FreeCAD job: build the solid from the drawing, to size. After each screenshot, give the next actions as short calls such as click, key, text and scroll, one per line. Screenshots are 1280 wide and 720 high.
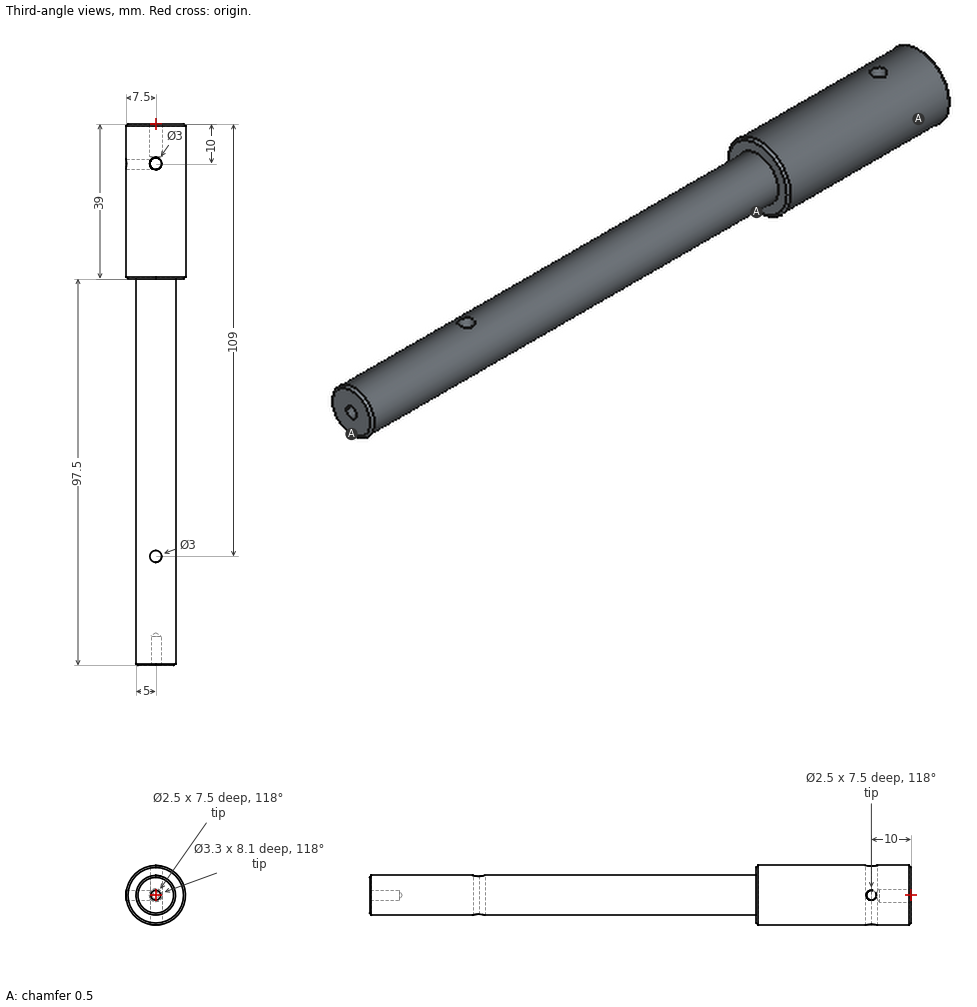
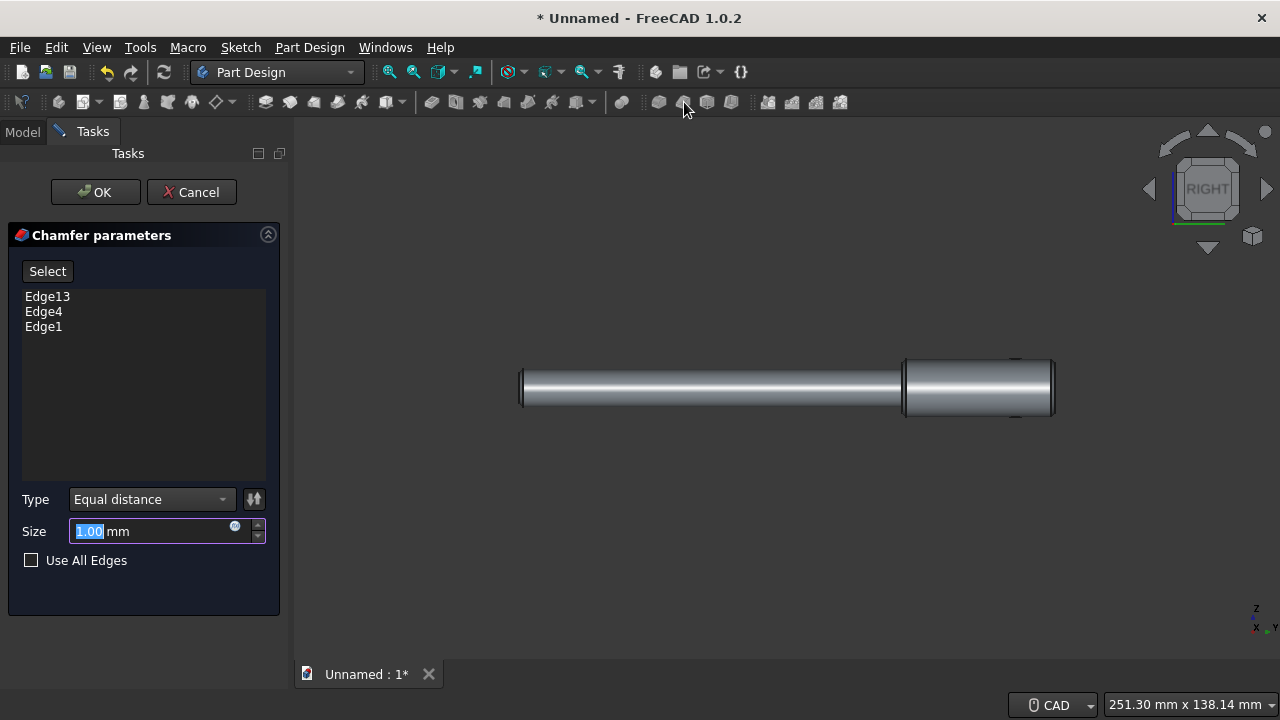
text(0.5)
key(Tab)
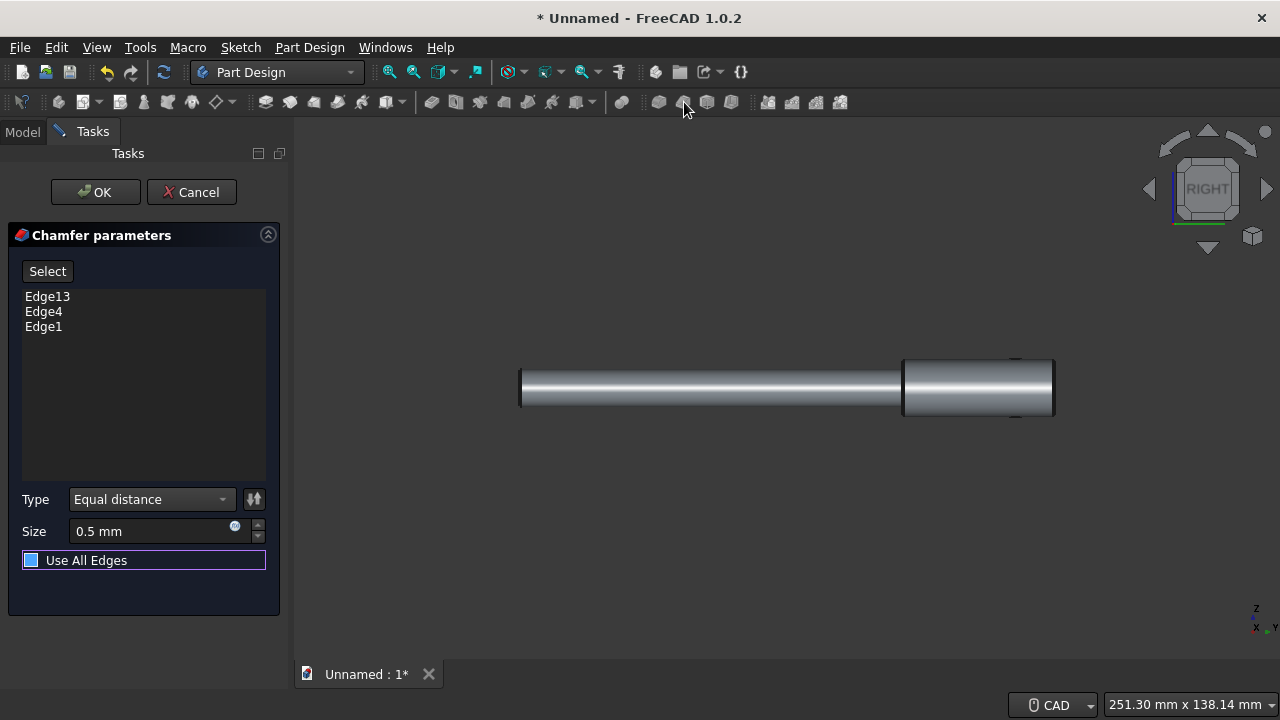
click(96, 192)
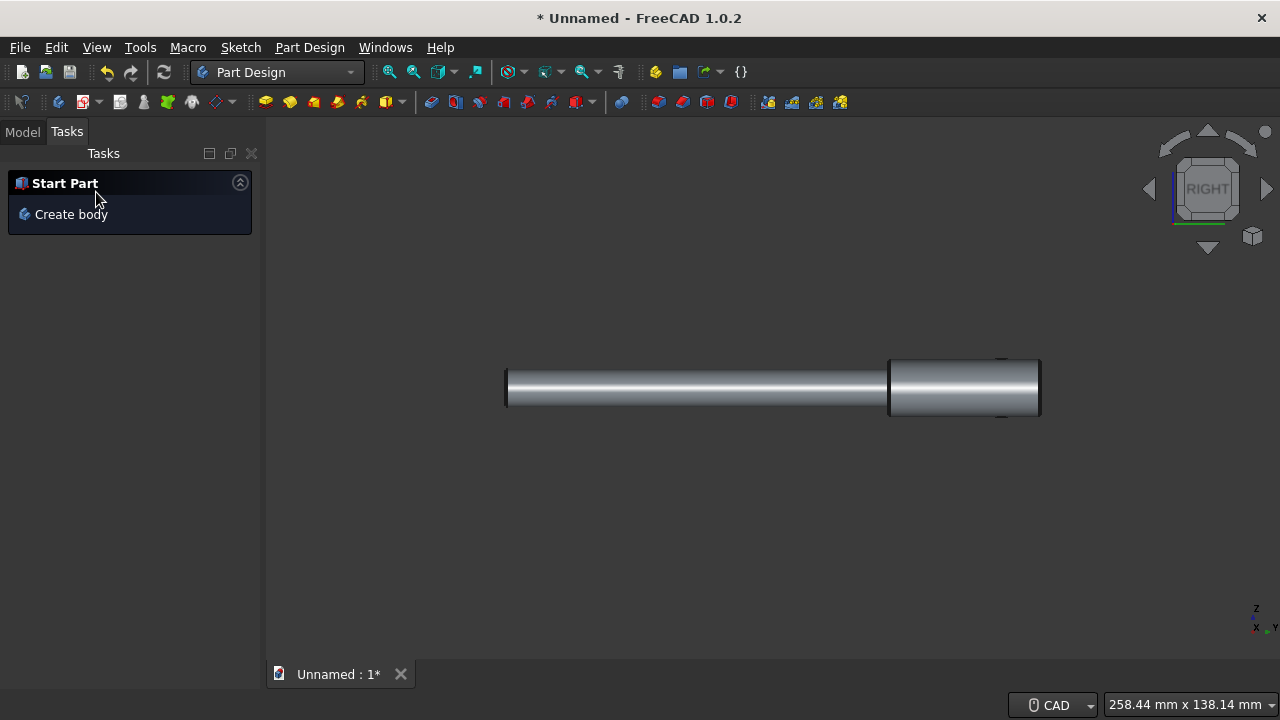
click(23, 131)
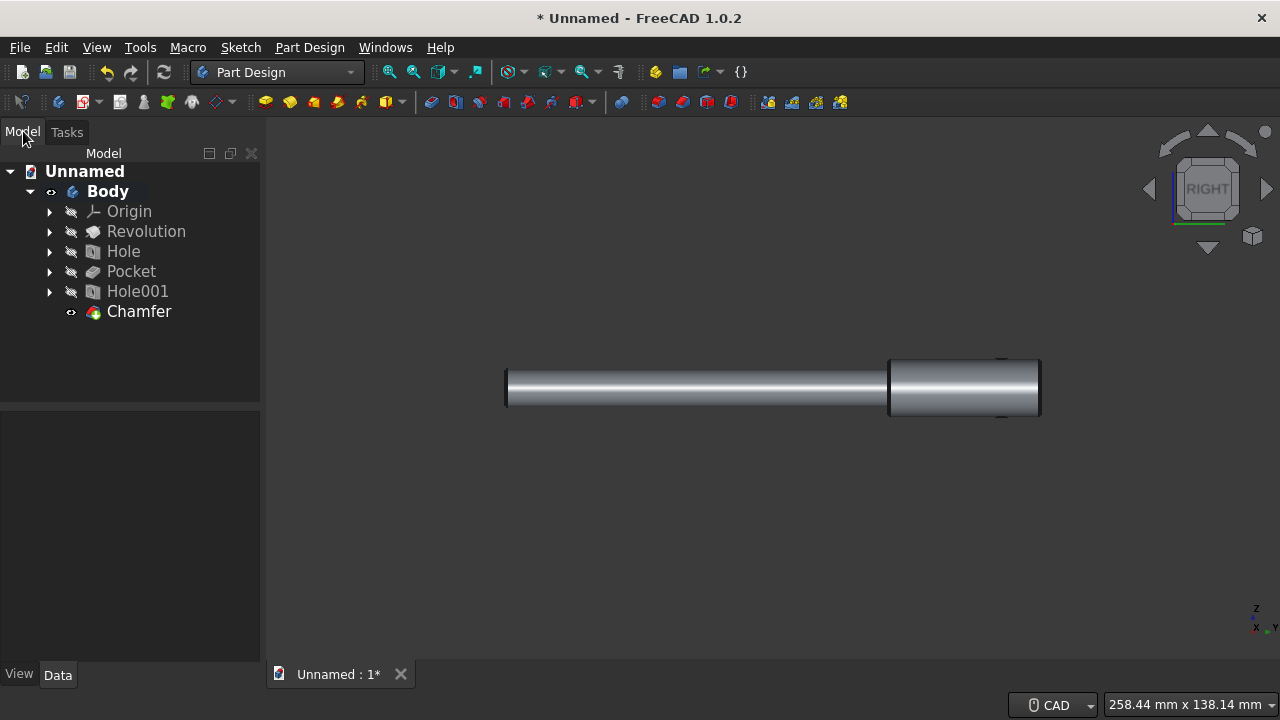
click(50, 212)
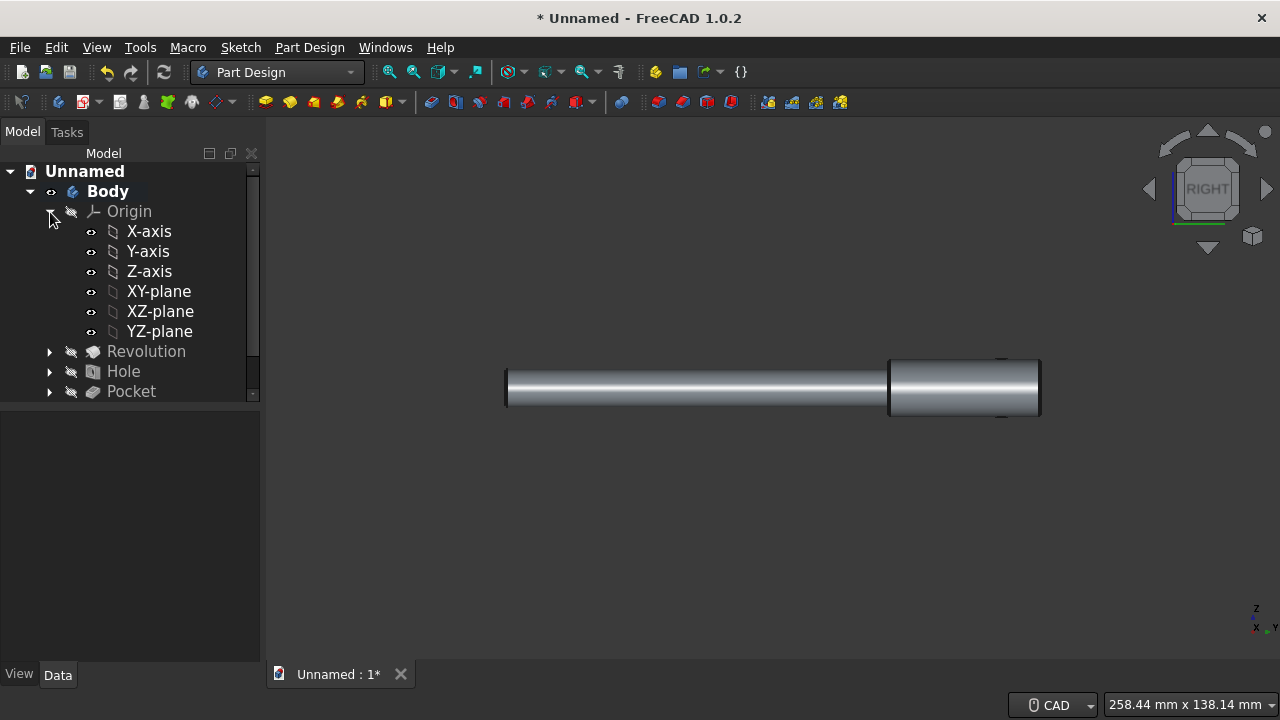
click(136, 332)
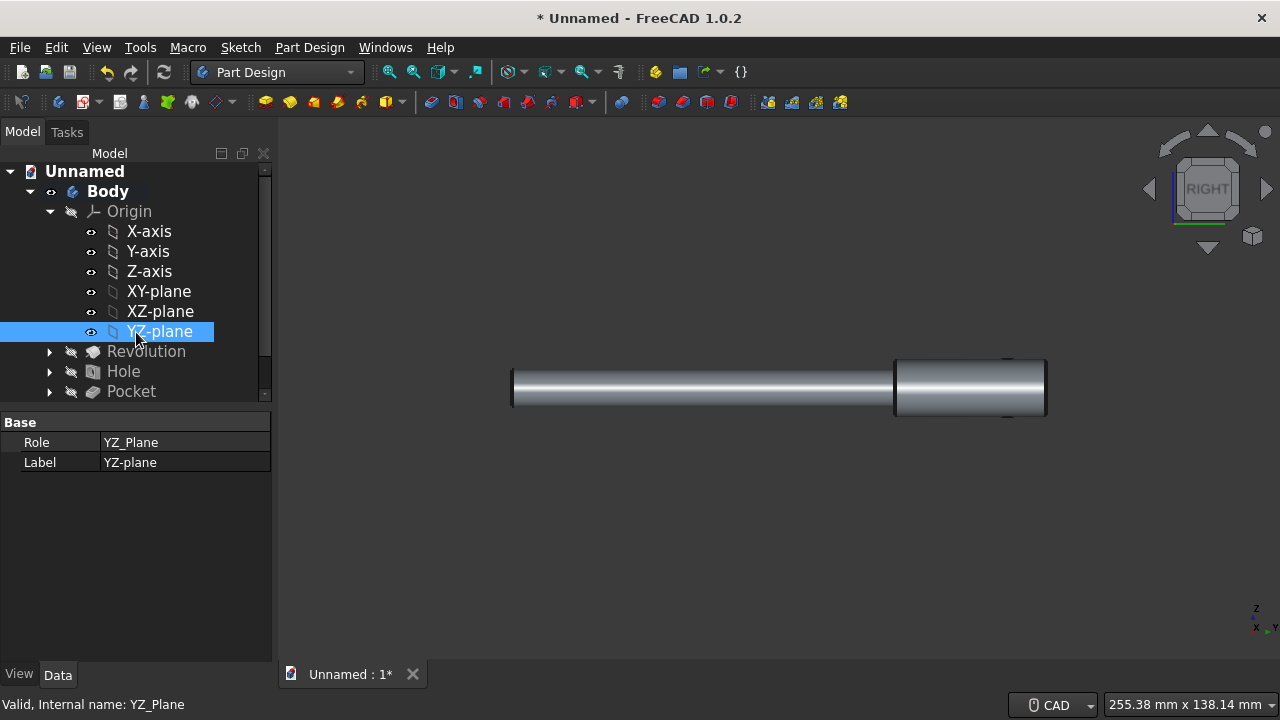
click(216, 102)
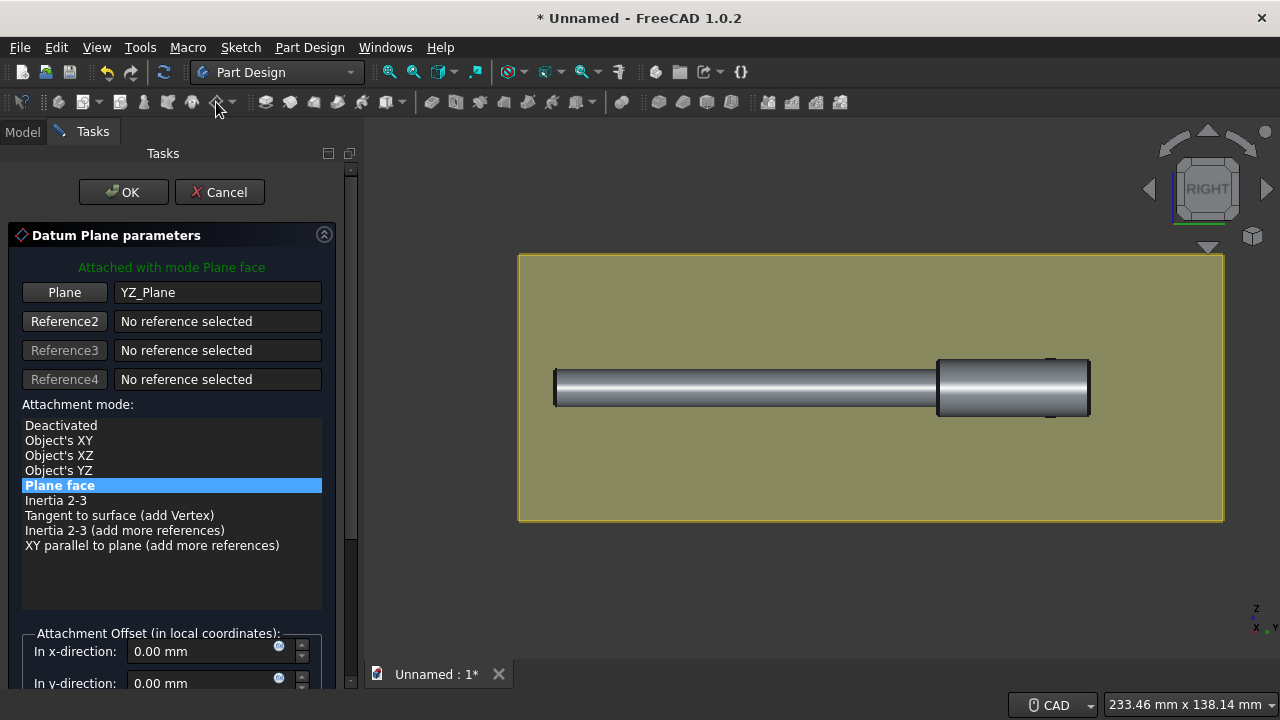
scroll(351, 426, down, 2)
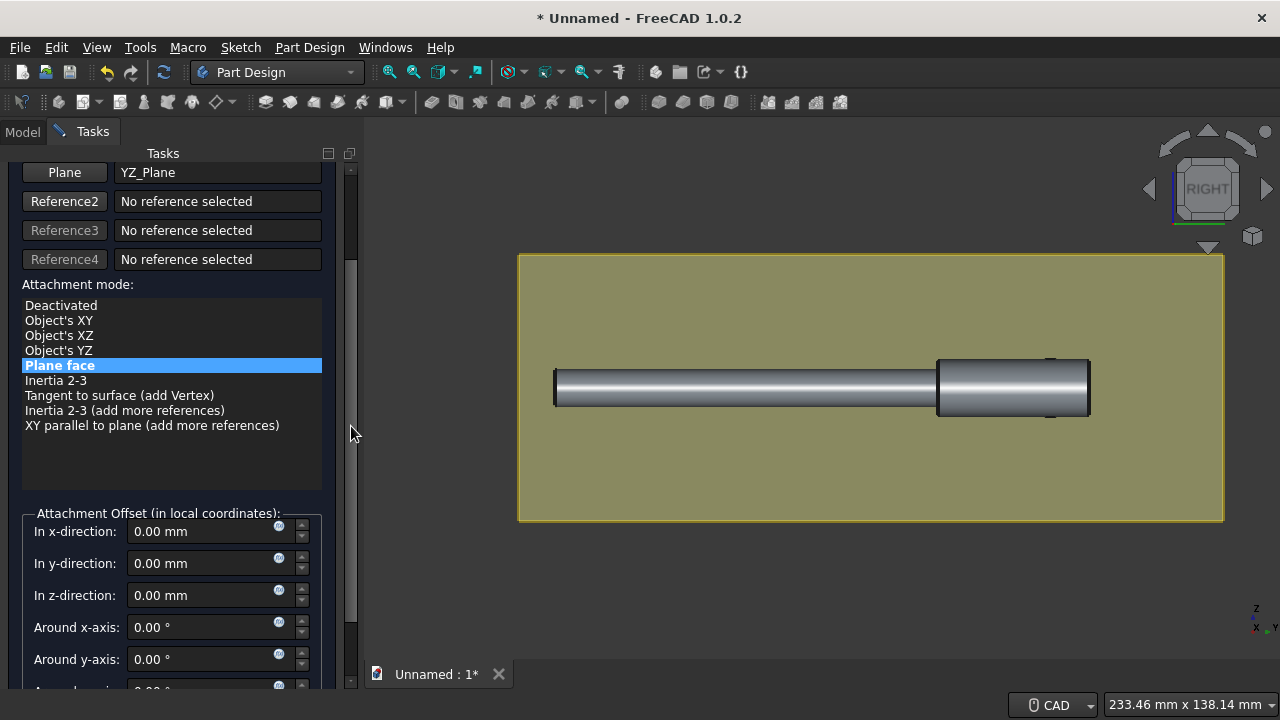
triple_click(210, 595)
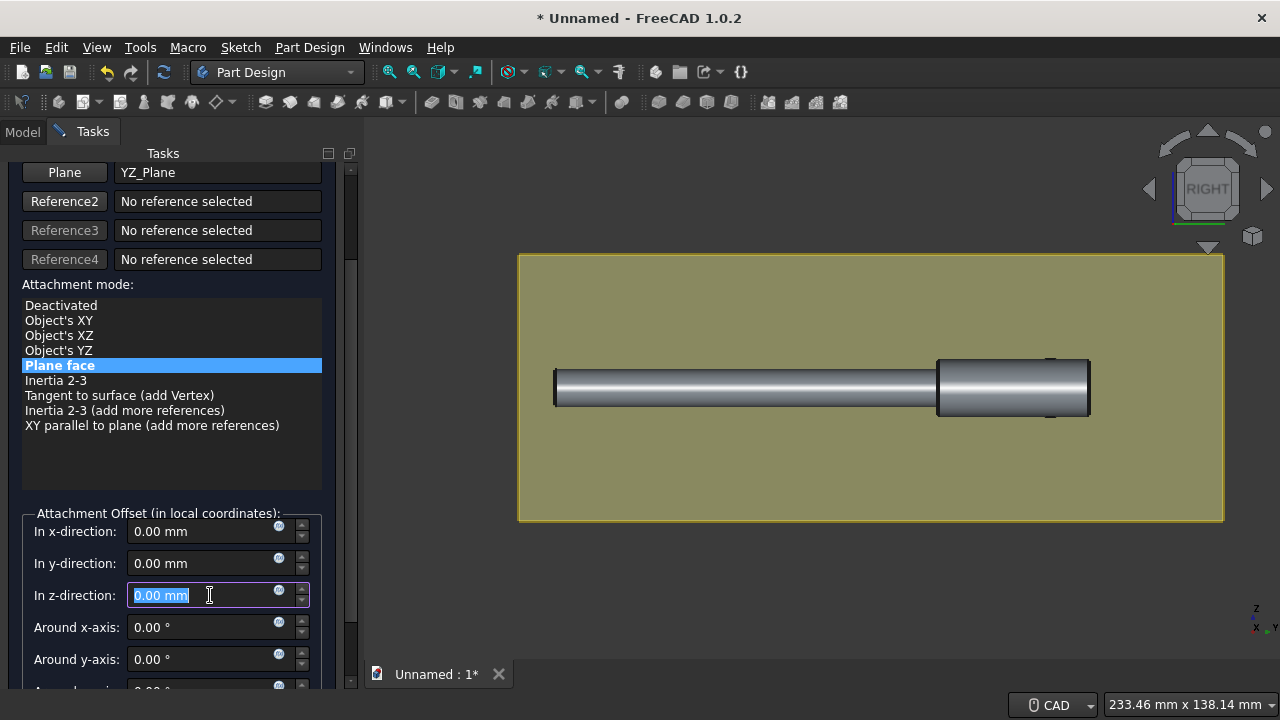
text(-7.5)
key(Tab)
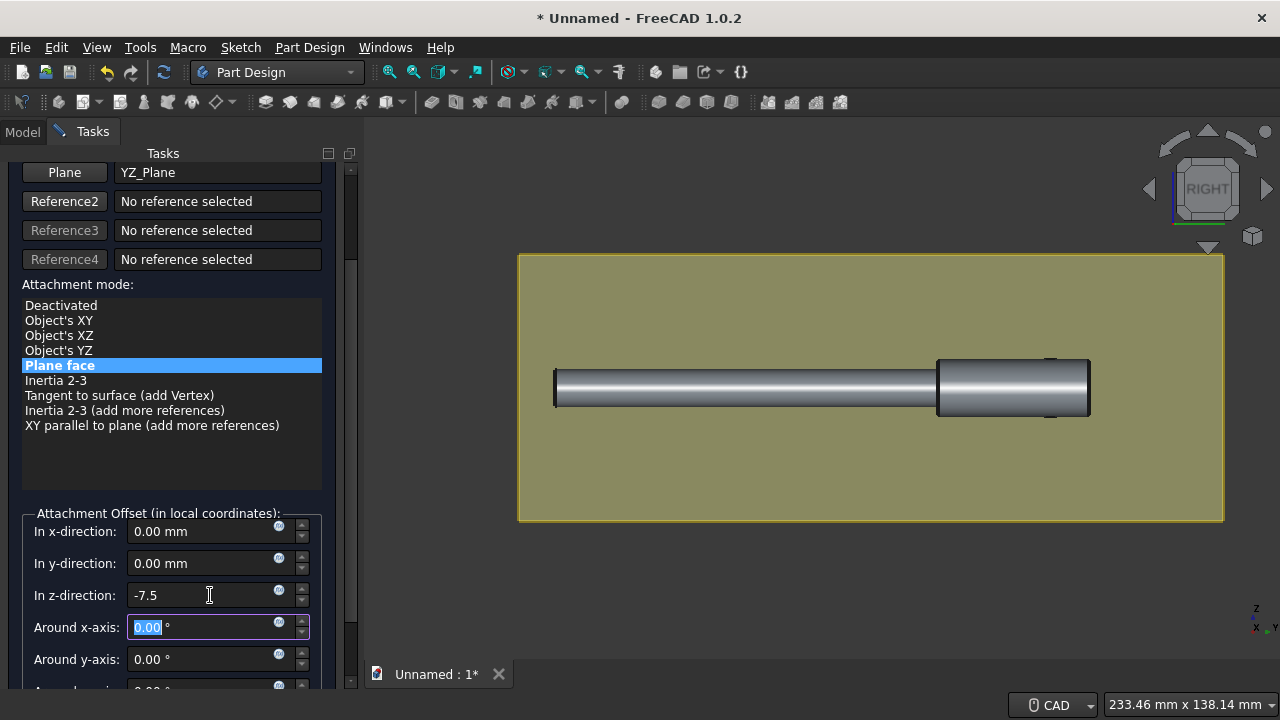
scroll(351, 426, up, 3)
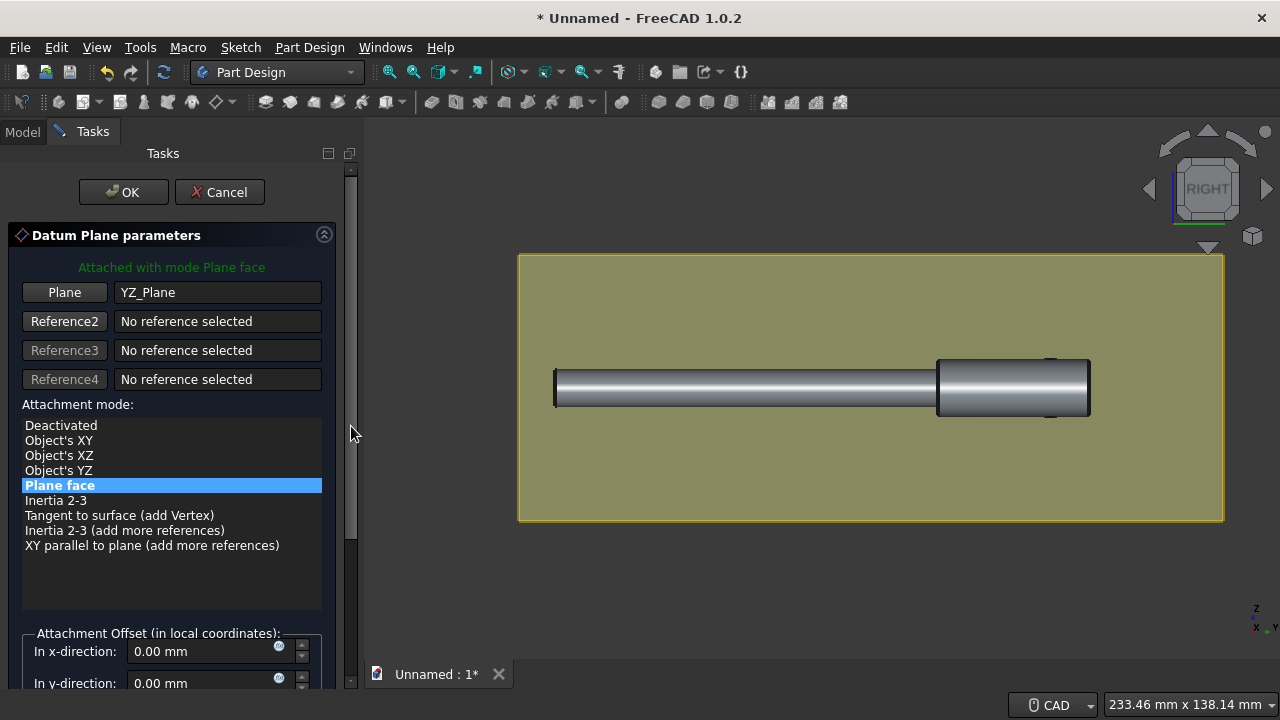
click(124, 192)